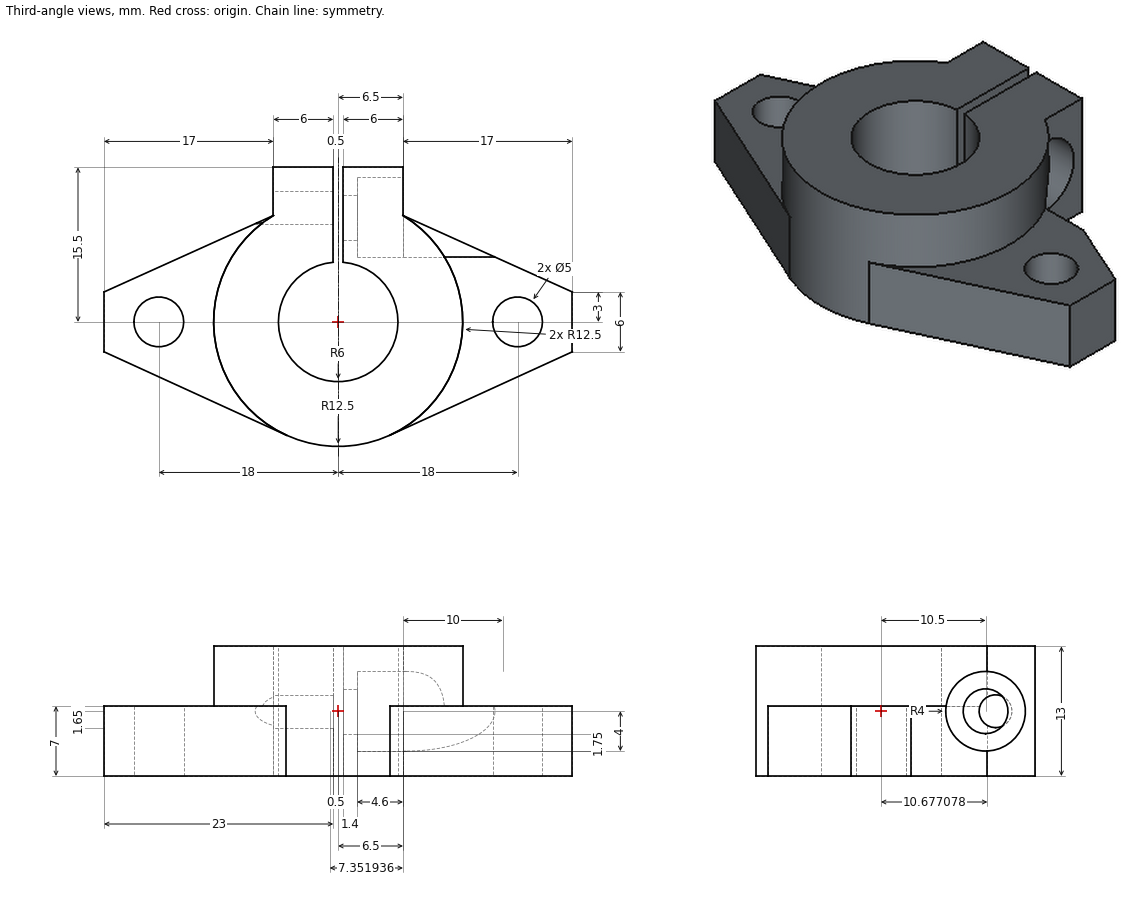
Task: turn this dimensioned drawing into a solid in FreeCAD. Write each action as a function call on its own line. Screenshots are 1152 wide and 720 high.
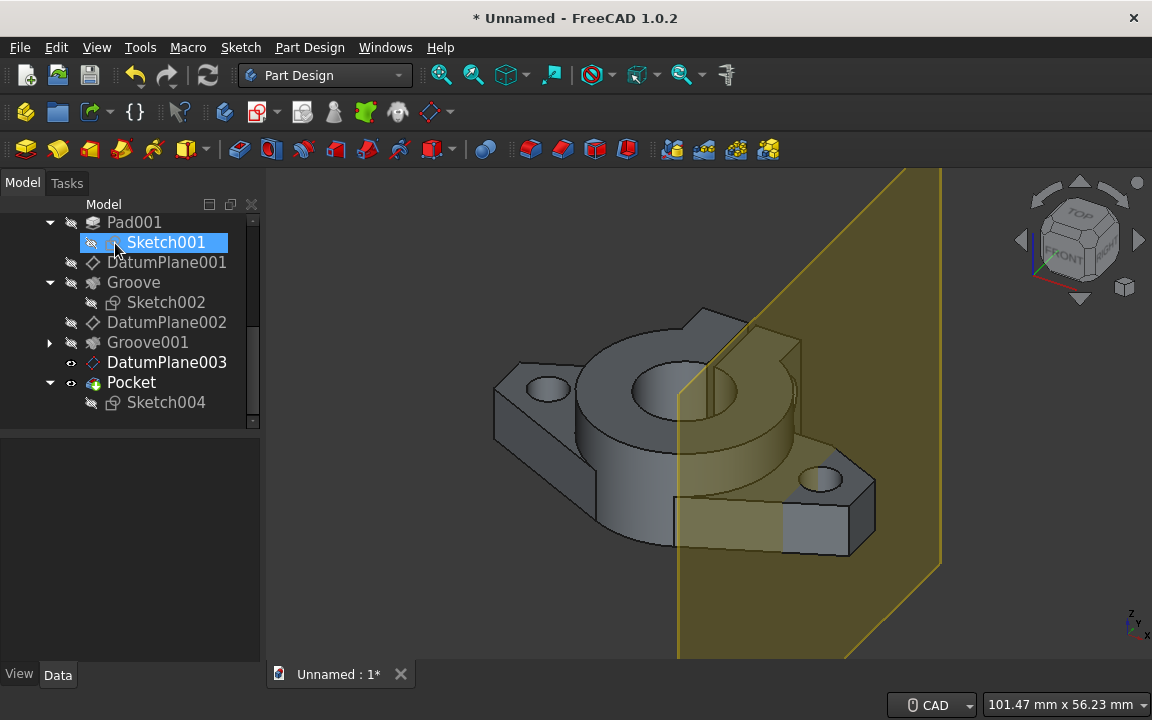
click(116, 363)
key(space)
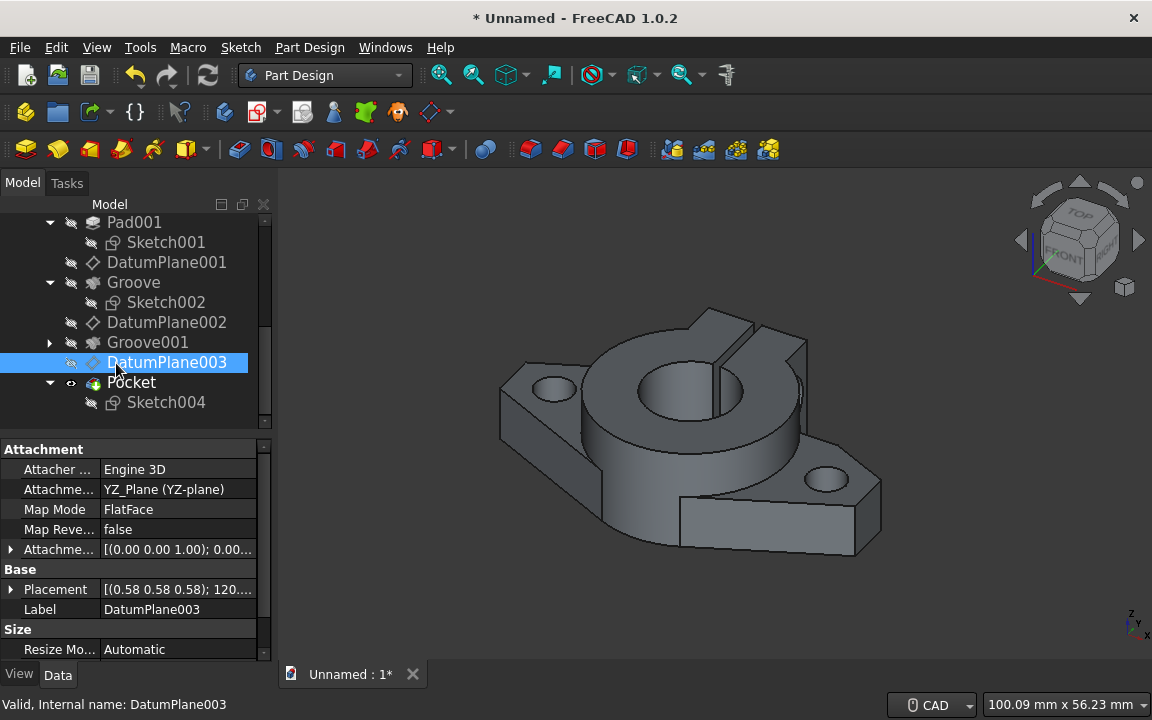
key(0)